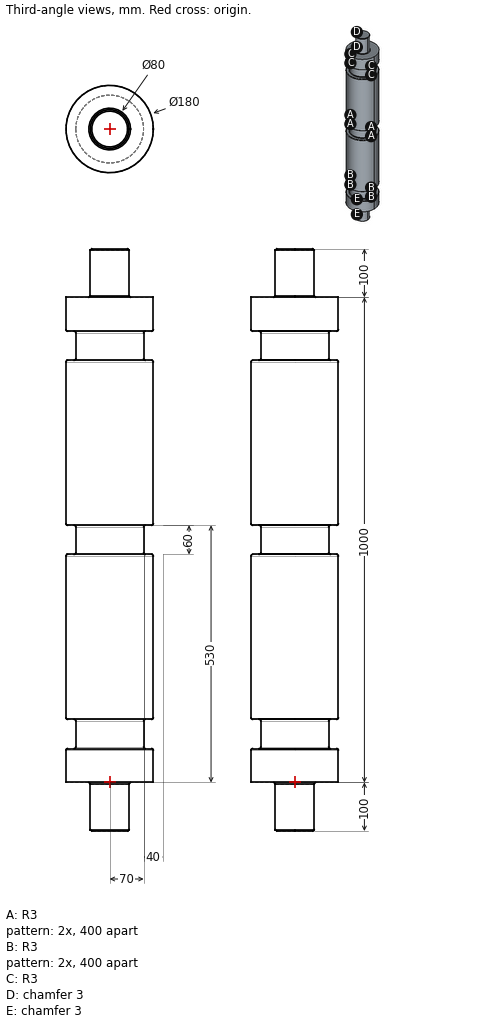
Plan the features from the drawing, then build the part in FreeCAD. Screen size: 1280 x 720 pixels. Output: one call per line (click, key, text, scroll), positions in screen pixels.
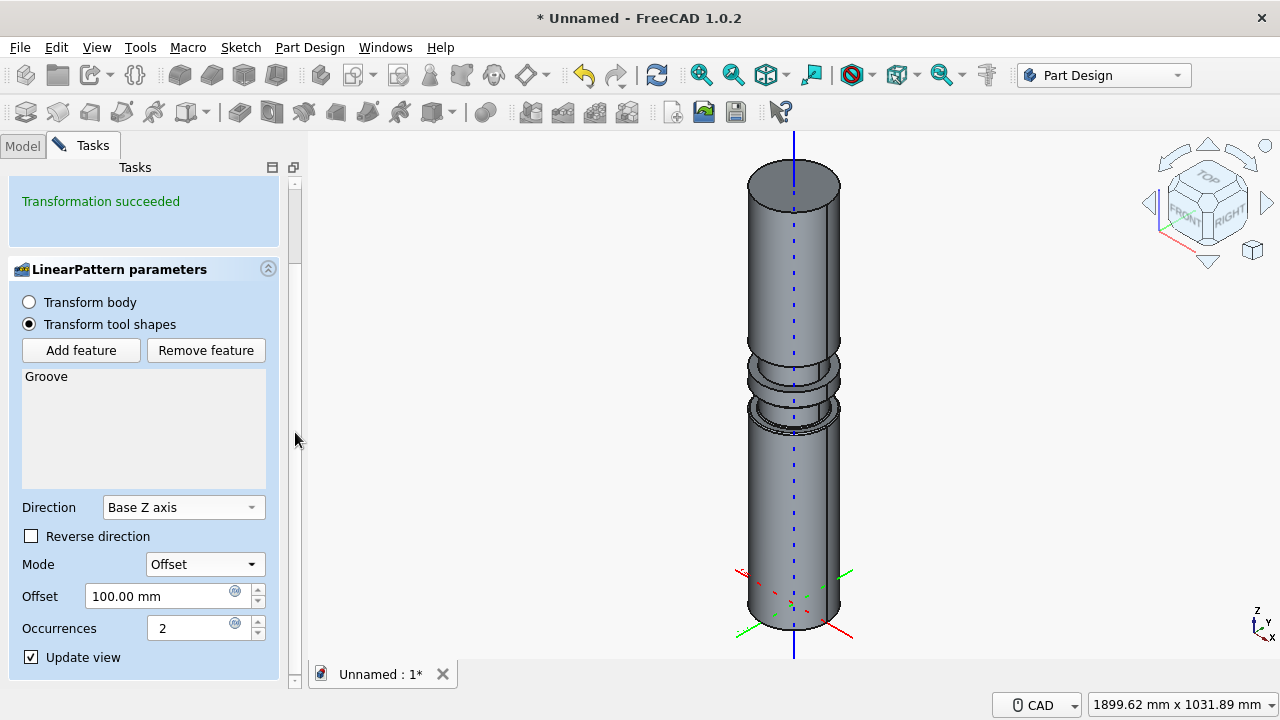
triple_click(168, 596)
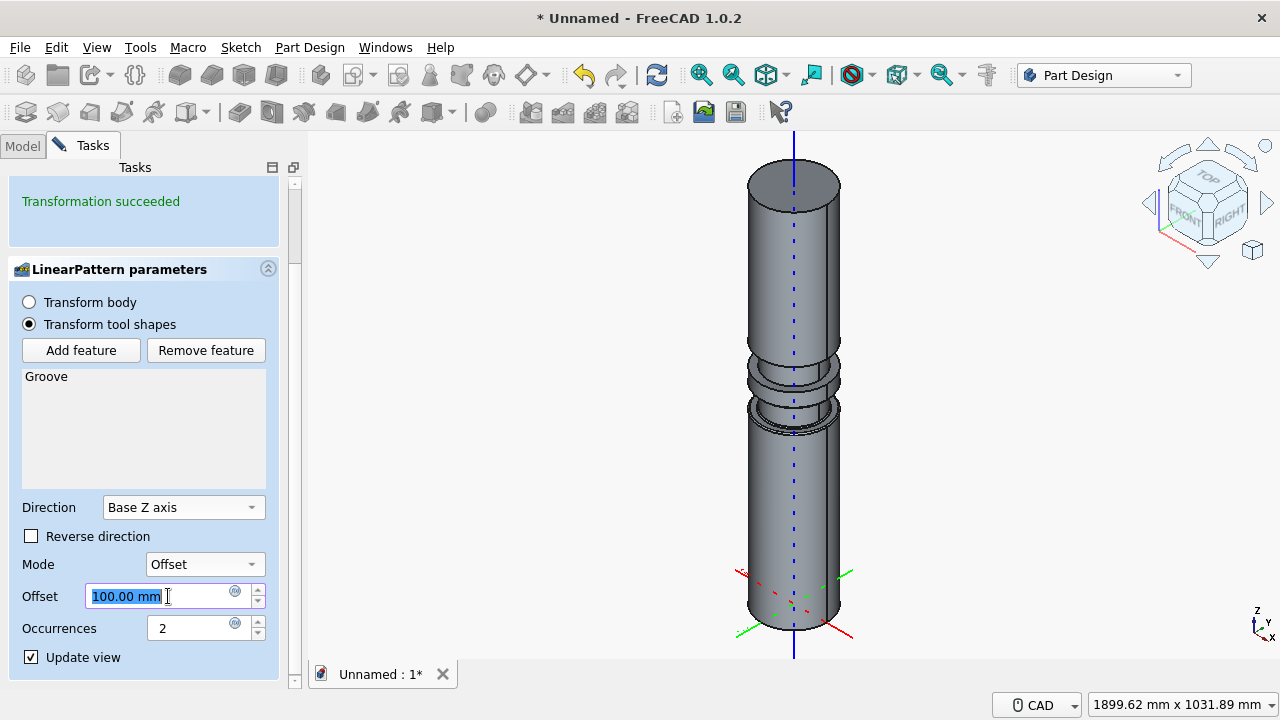
text(400)
key(Tab)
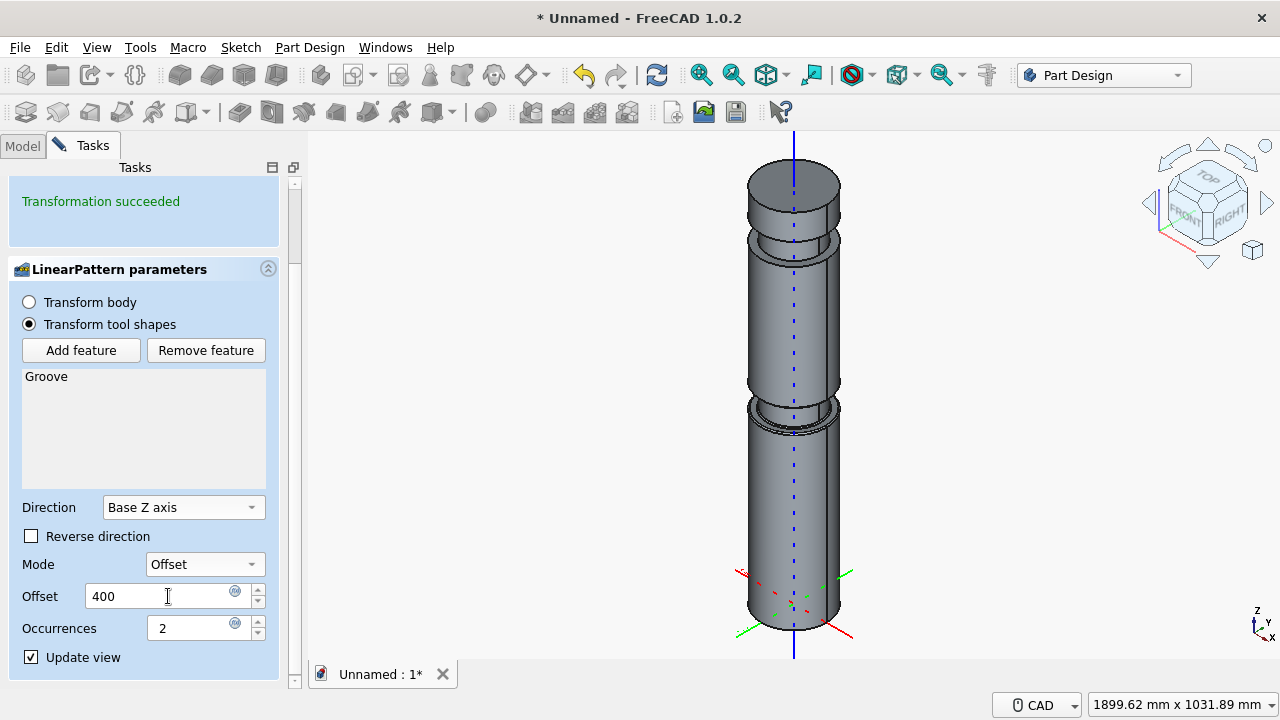
triple_click(198, 628)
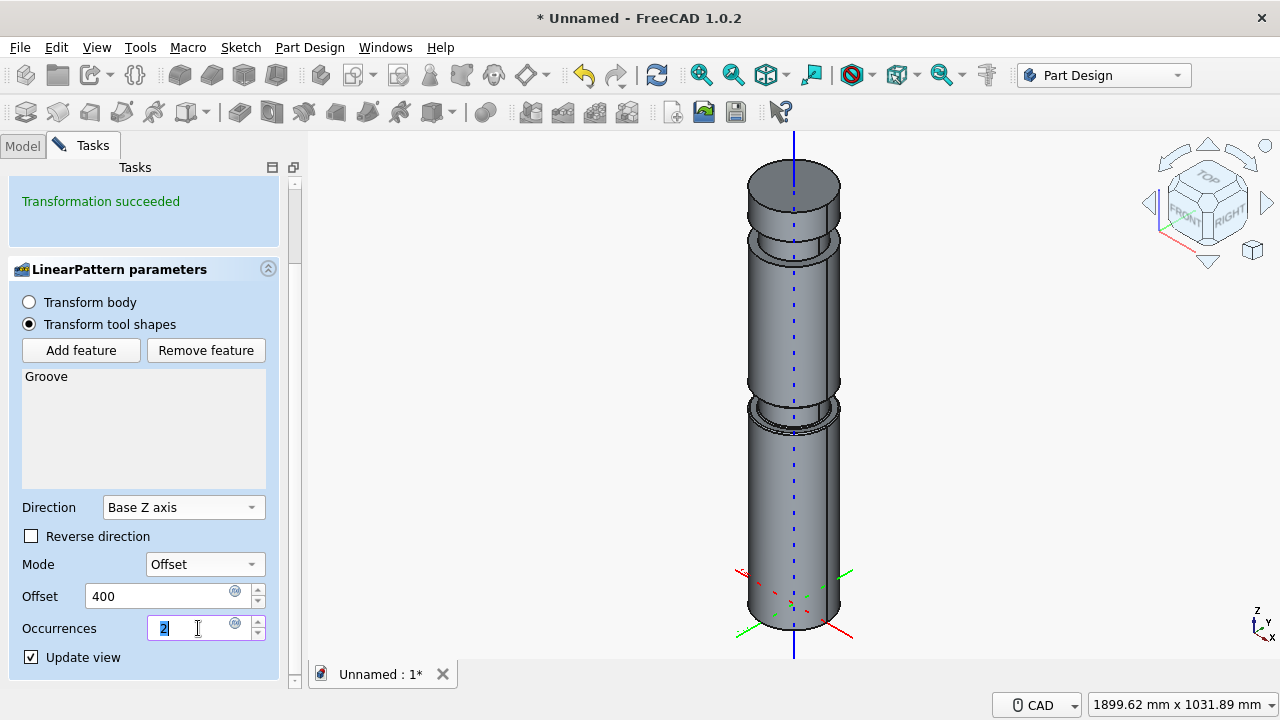
text(2)
key(Tab)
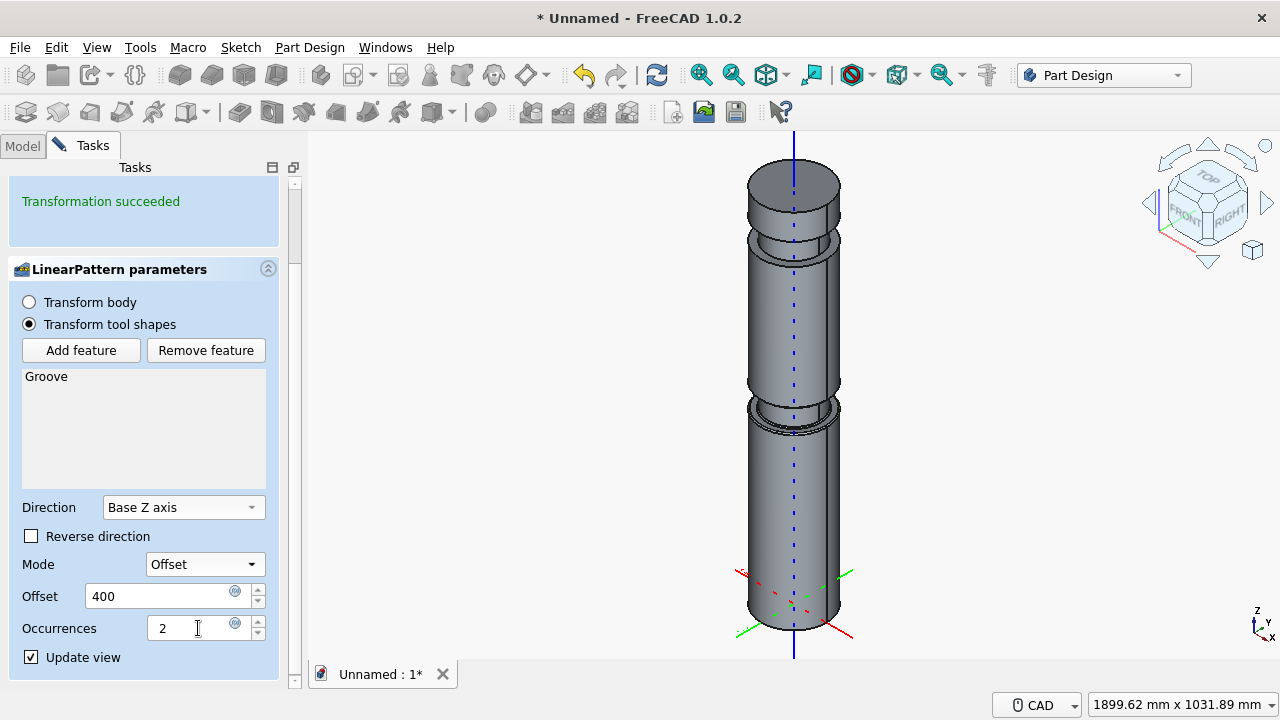
click(30, 536)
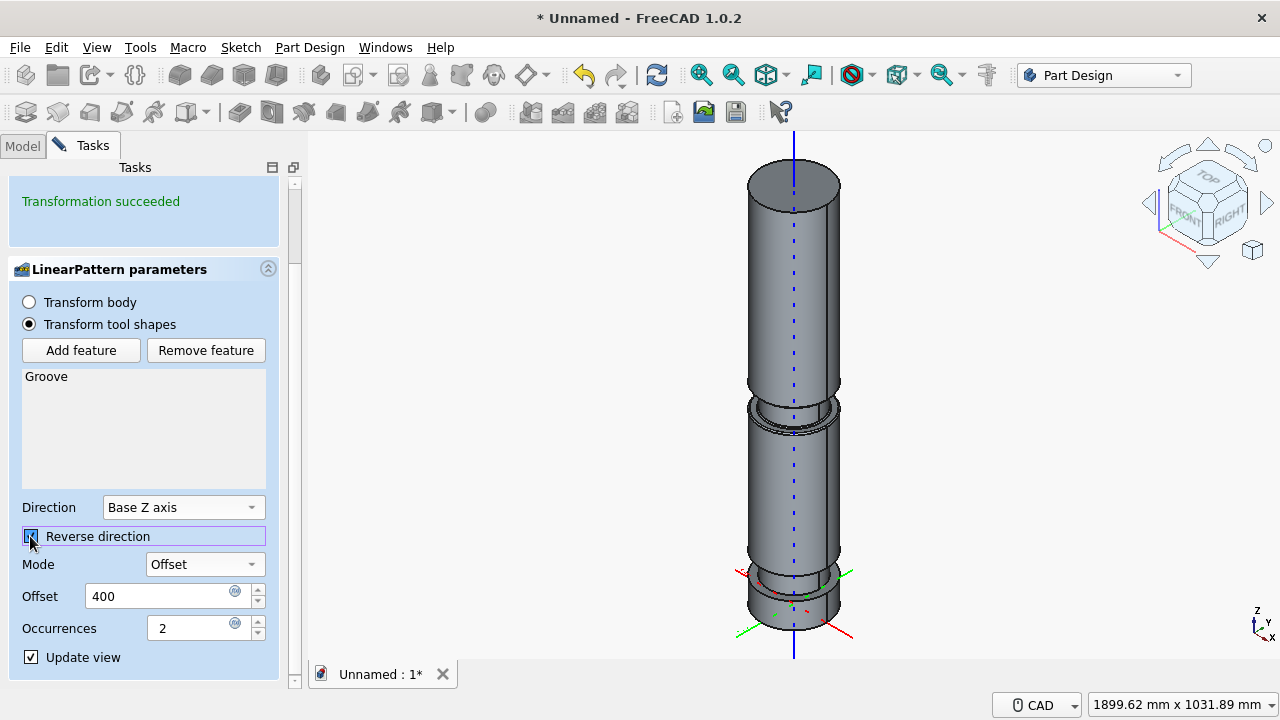
scroll(295, 432, up, 3)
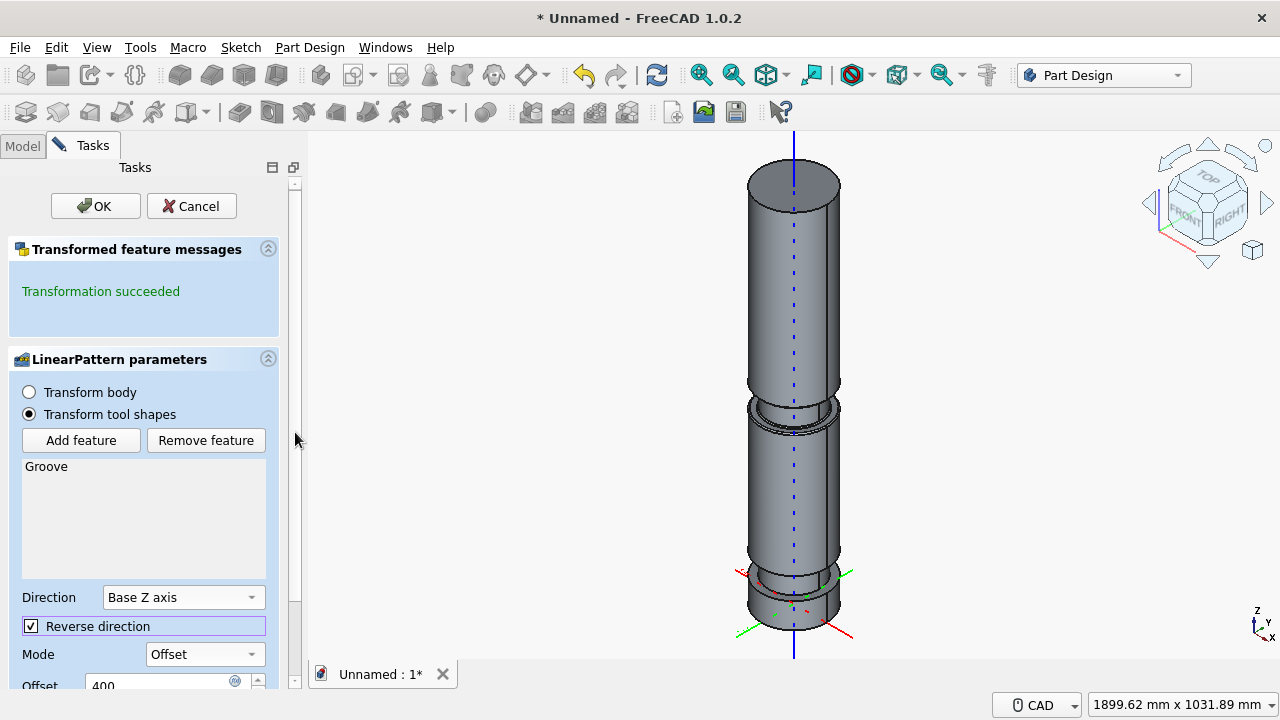
click(96, 206)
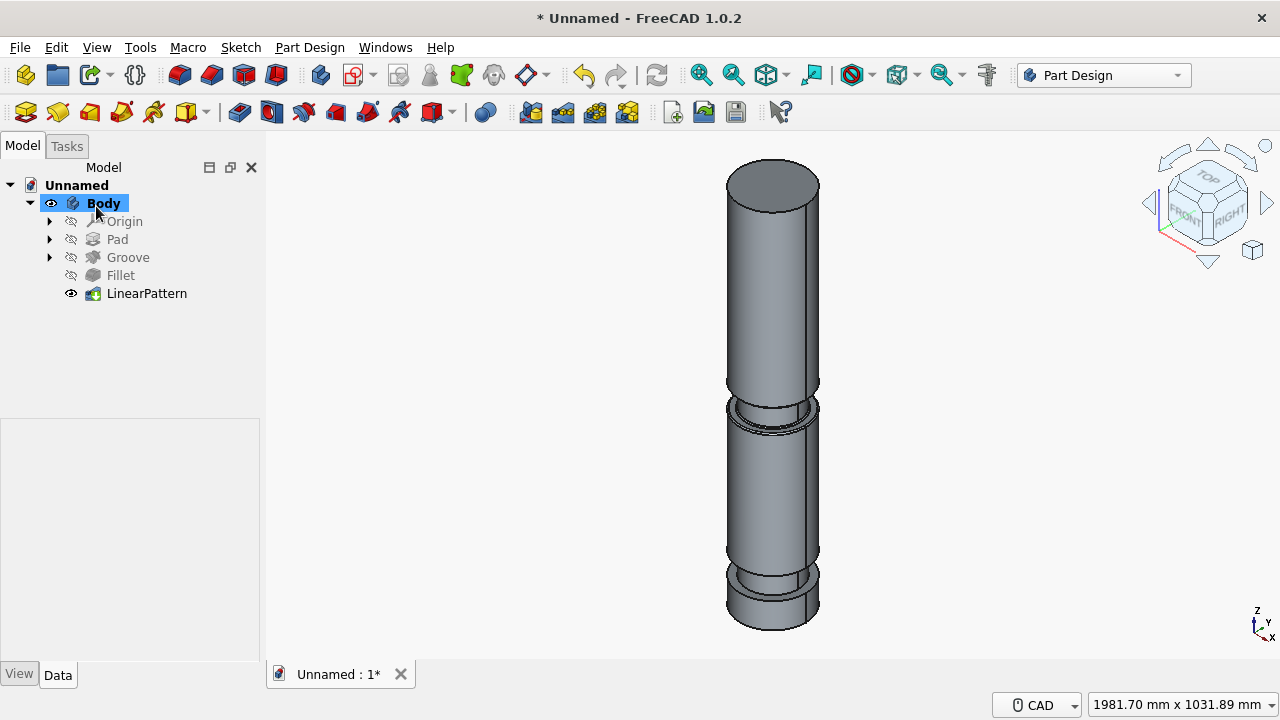
click(732, 561)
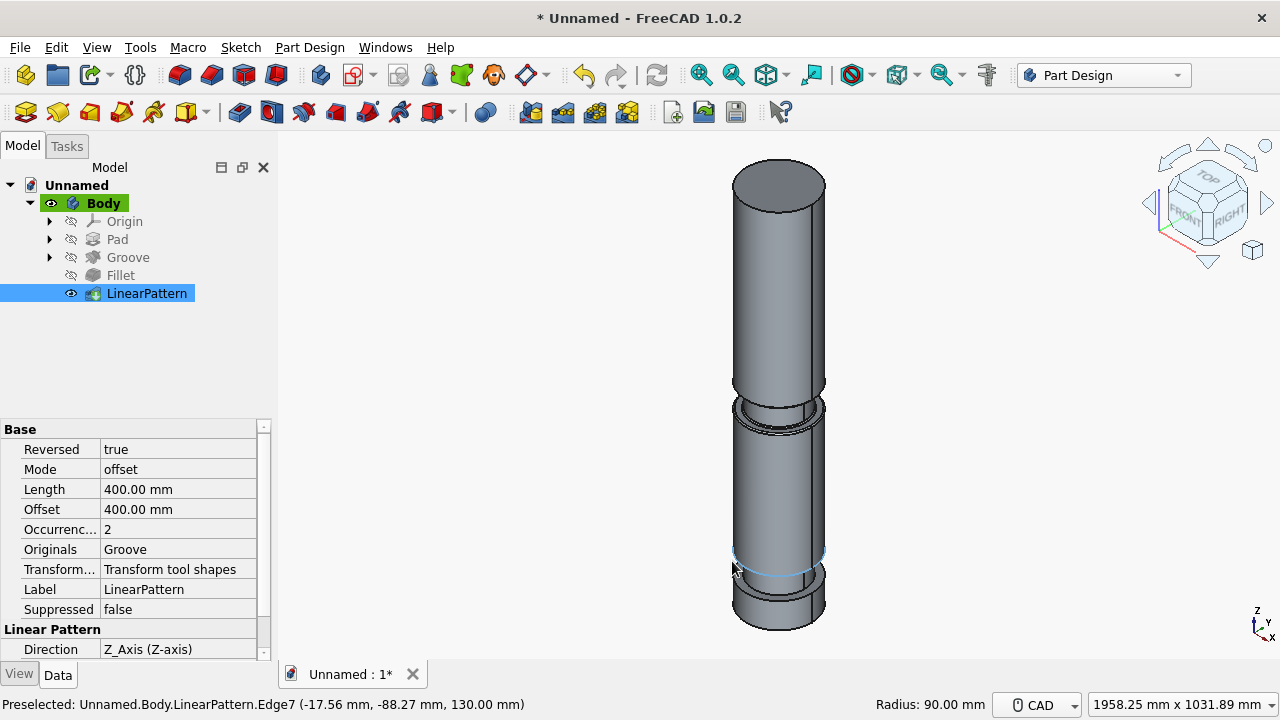
click(738, 586, ctrl)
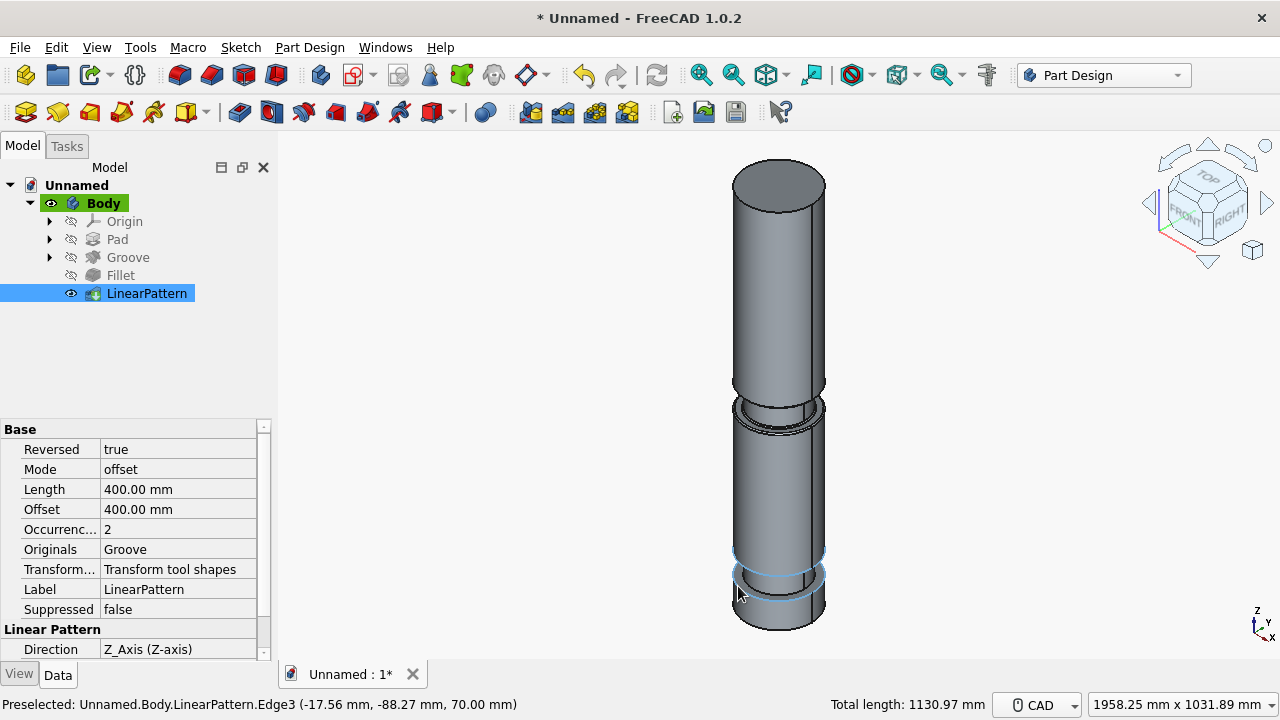
key(2)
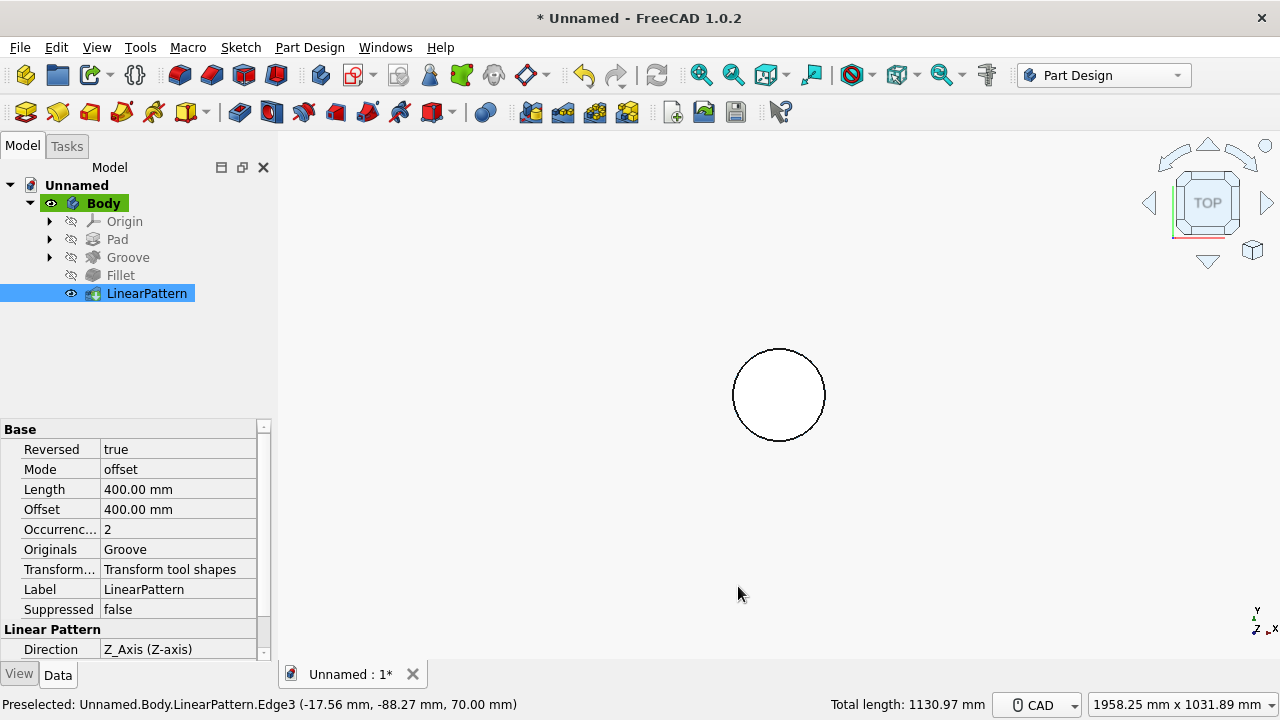
click(702, 76)